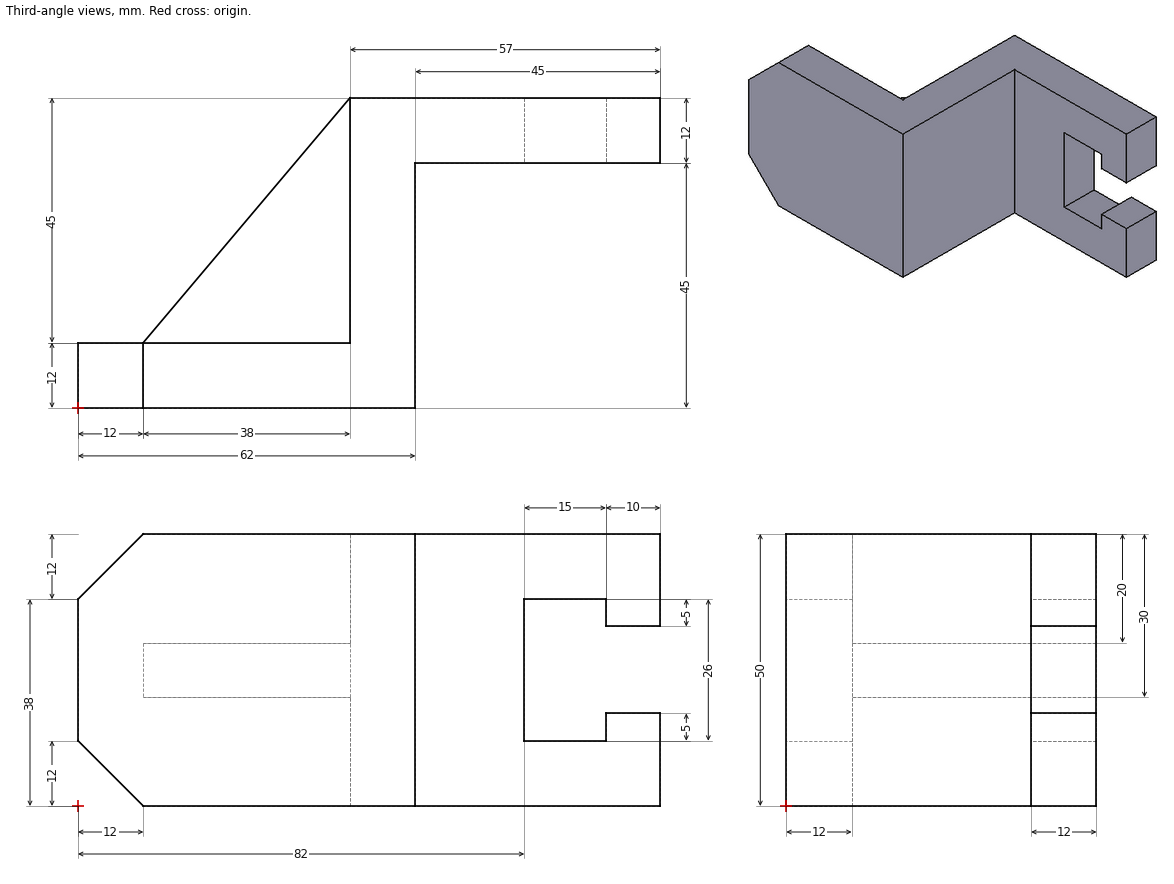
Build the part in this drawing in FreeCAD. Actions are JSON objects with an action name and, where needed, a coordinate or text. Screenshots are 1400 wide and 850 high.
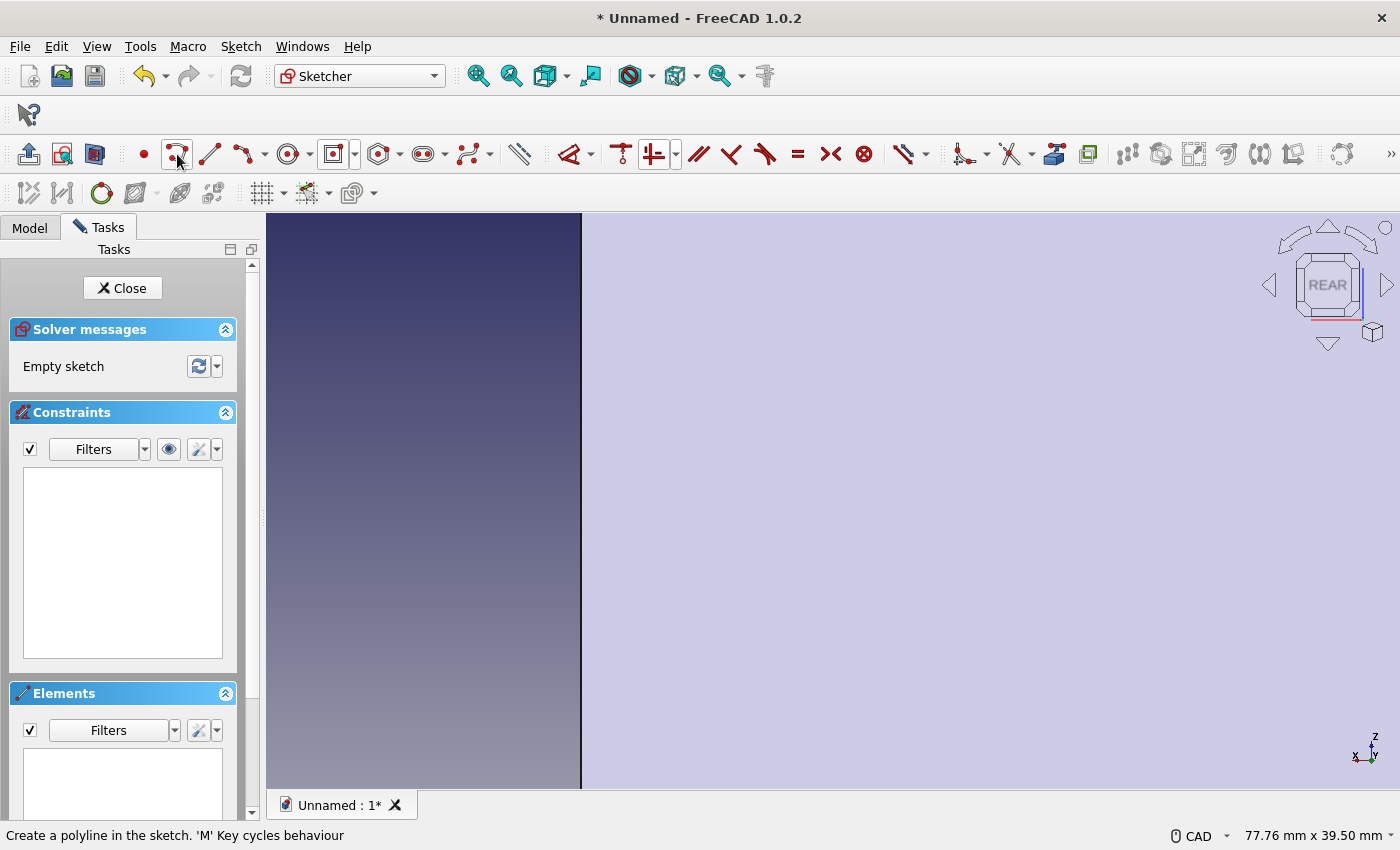
{"action": "left_click", "coordinate": [946, 689]}
{"action": "left_click", "coordinate": [946, 310]}
{"action": "left_click", "coordinate": [727, 310]}
{"action": "left_click", "coordinate": [727, 383]}
{"action": "left_click", "coordinate": [581, 383]}
{"action": "left_click", "coordinate": [581, 616]}
{"action": "left_click", "coordinate": [727, 616]}
{"action": "left_click", "coordinate": [727, 689]}
{"action": "left_click", "coordinate": [946, 690]}
{"action": "key", "text": "Escape"}
{"action": "key", "text": "Escape"}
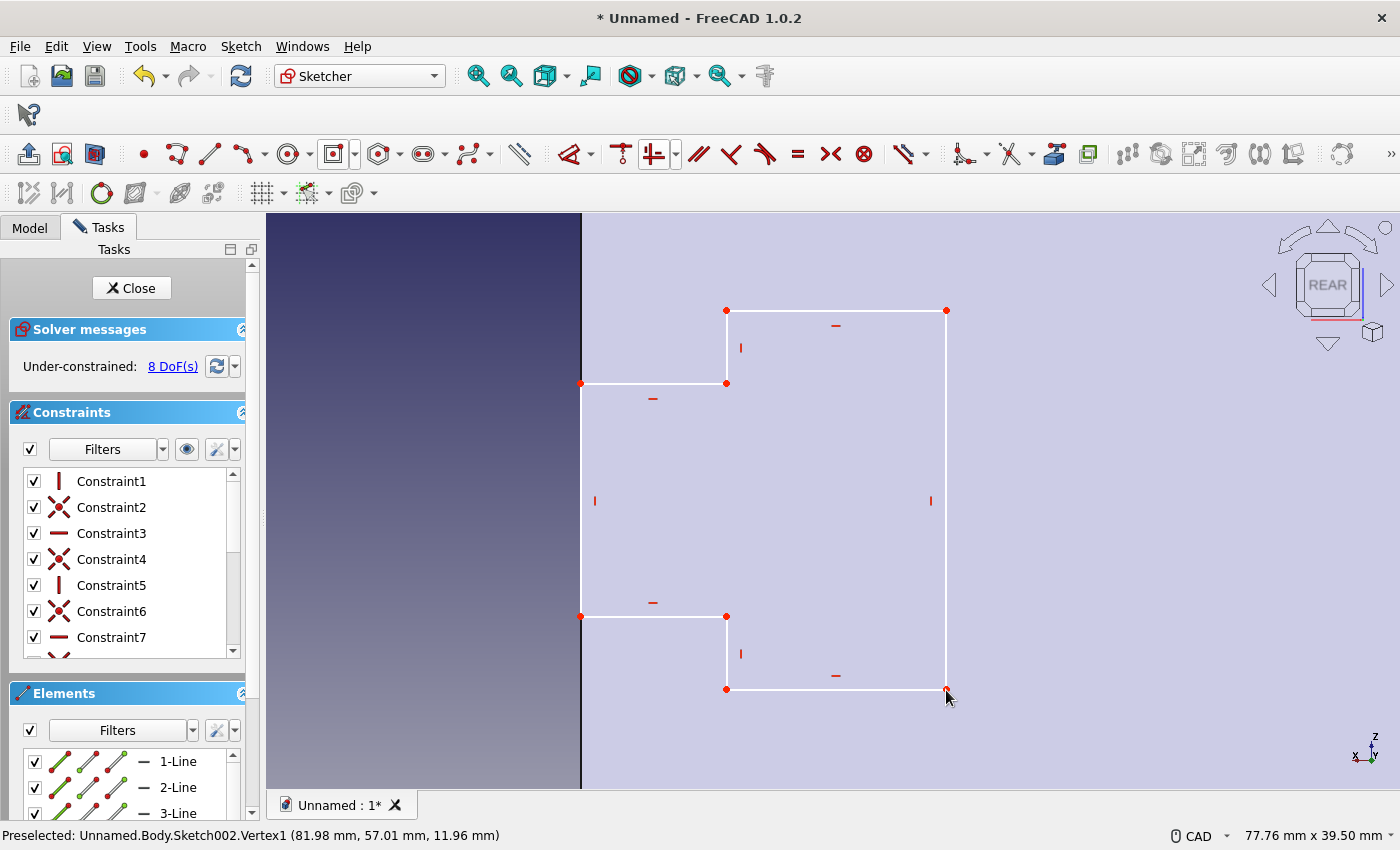
{"action": "left_click", "coordinate": [568, 154]}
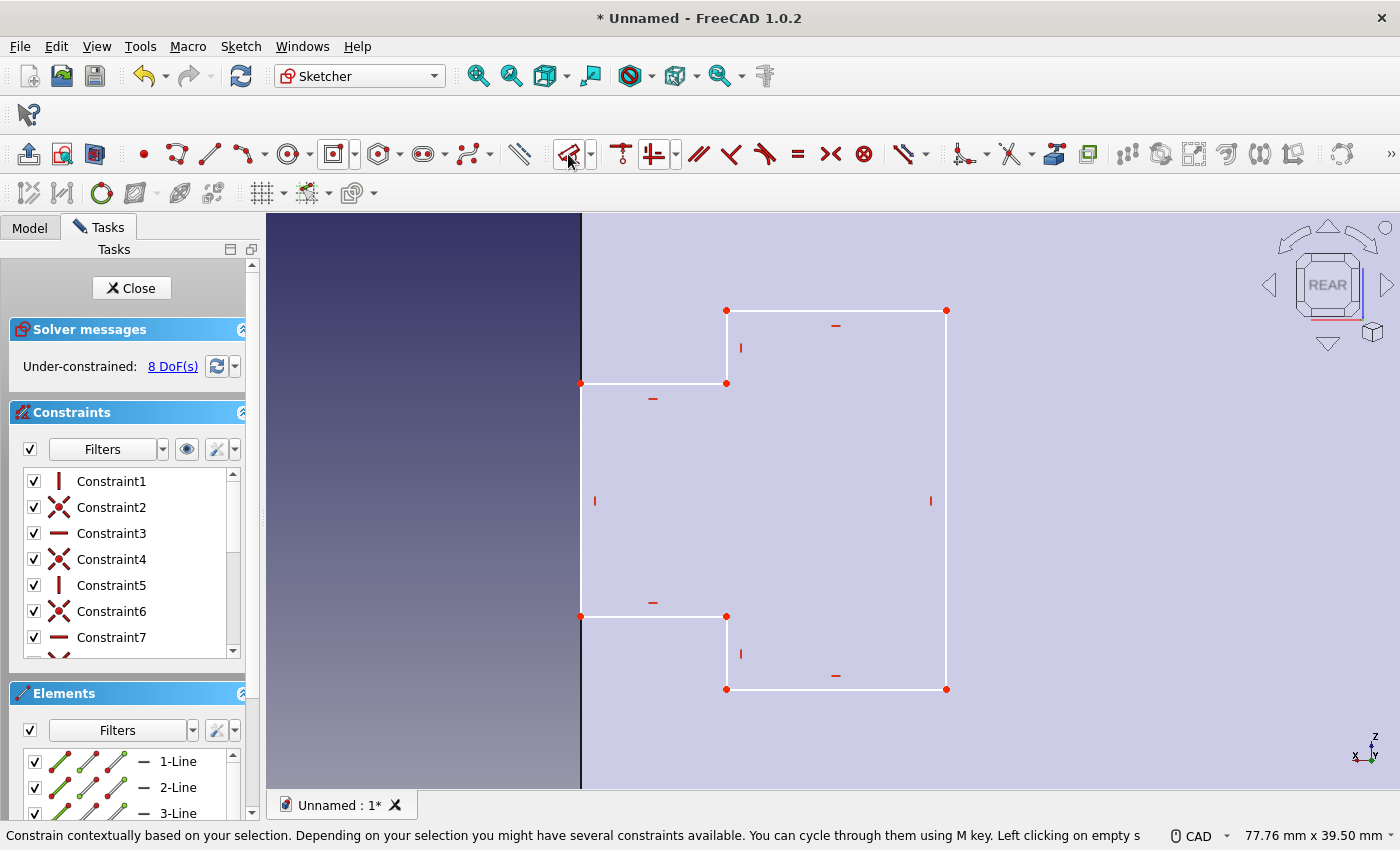
{"action": "left_click", "coordinate": [727, 333]}
{"action": "left_click", "coordinate": [693, 347]}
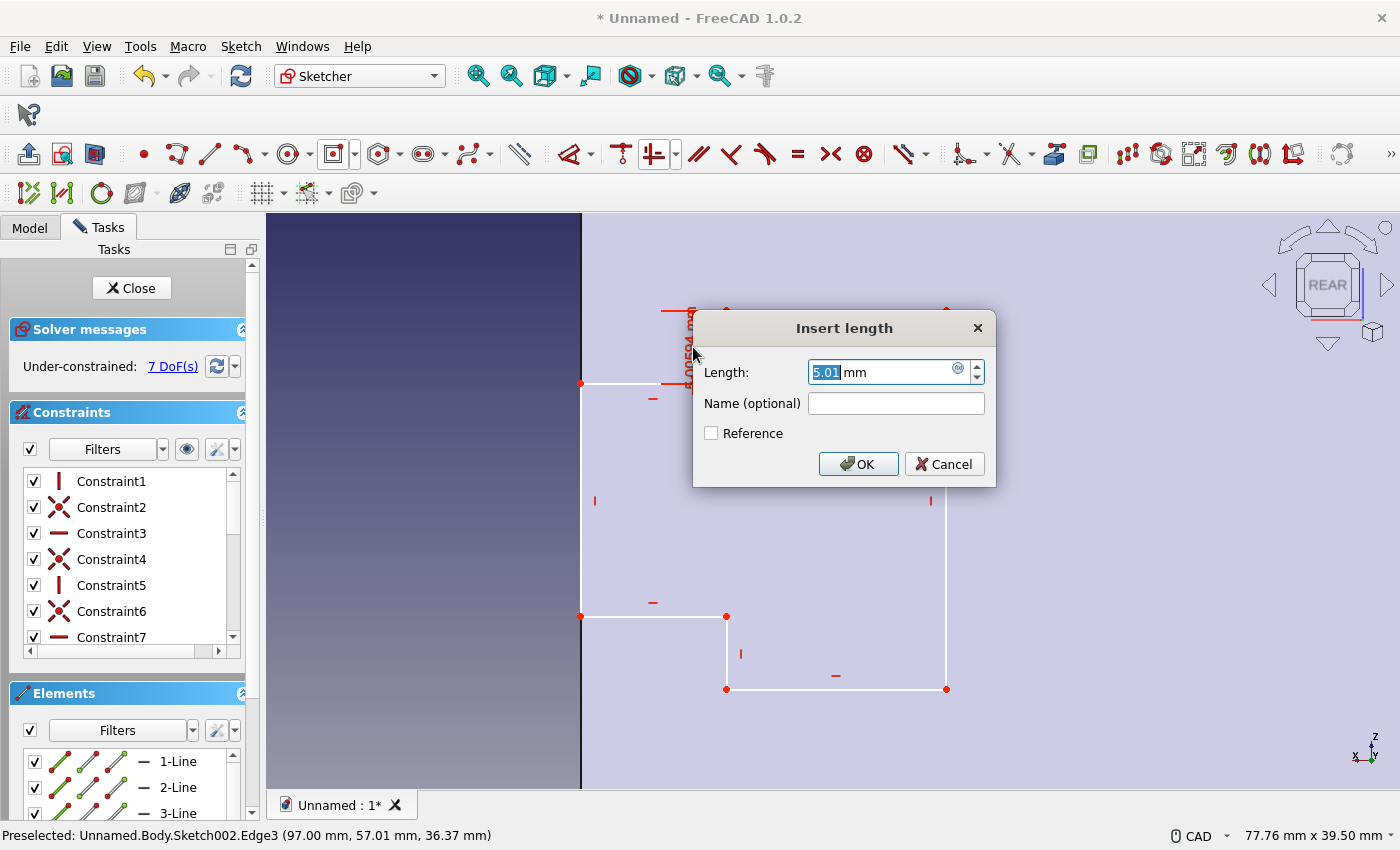
{"action": "type", "text": "5"}
{"action": "key", "text": "Return"}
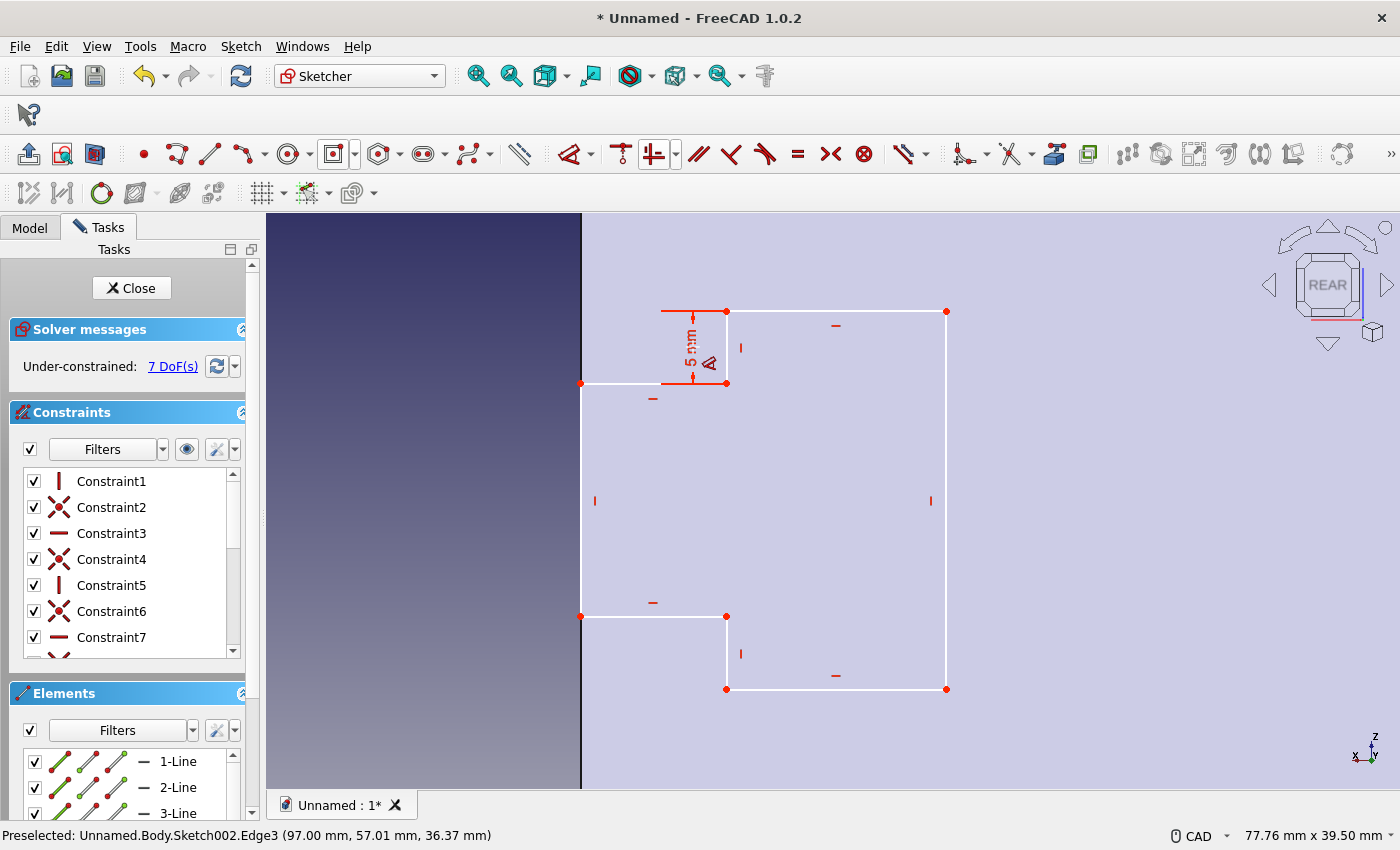
{"action": "left_click", "coordinate": [727, 639]}
{"action": "left_click", "coordinate": [693, 653]}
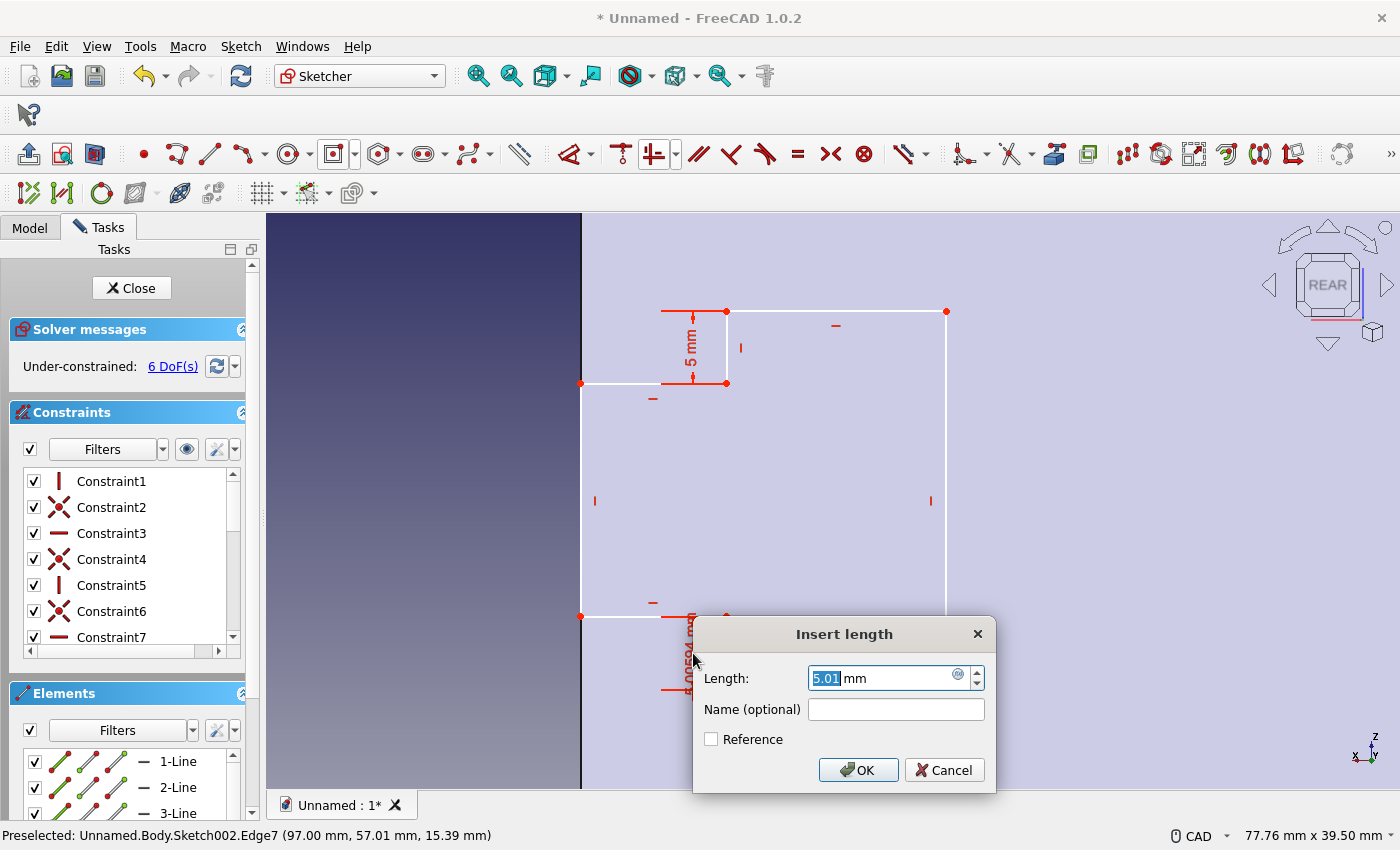
{"action": "type", "text": "5"}
{"action": "key", "text": "Return"}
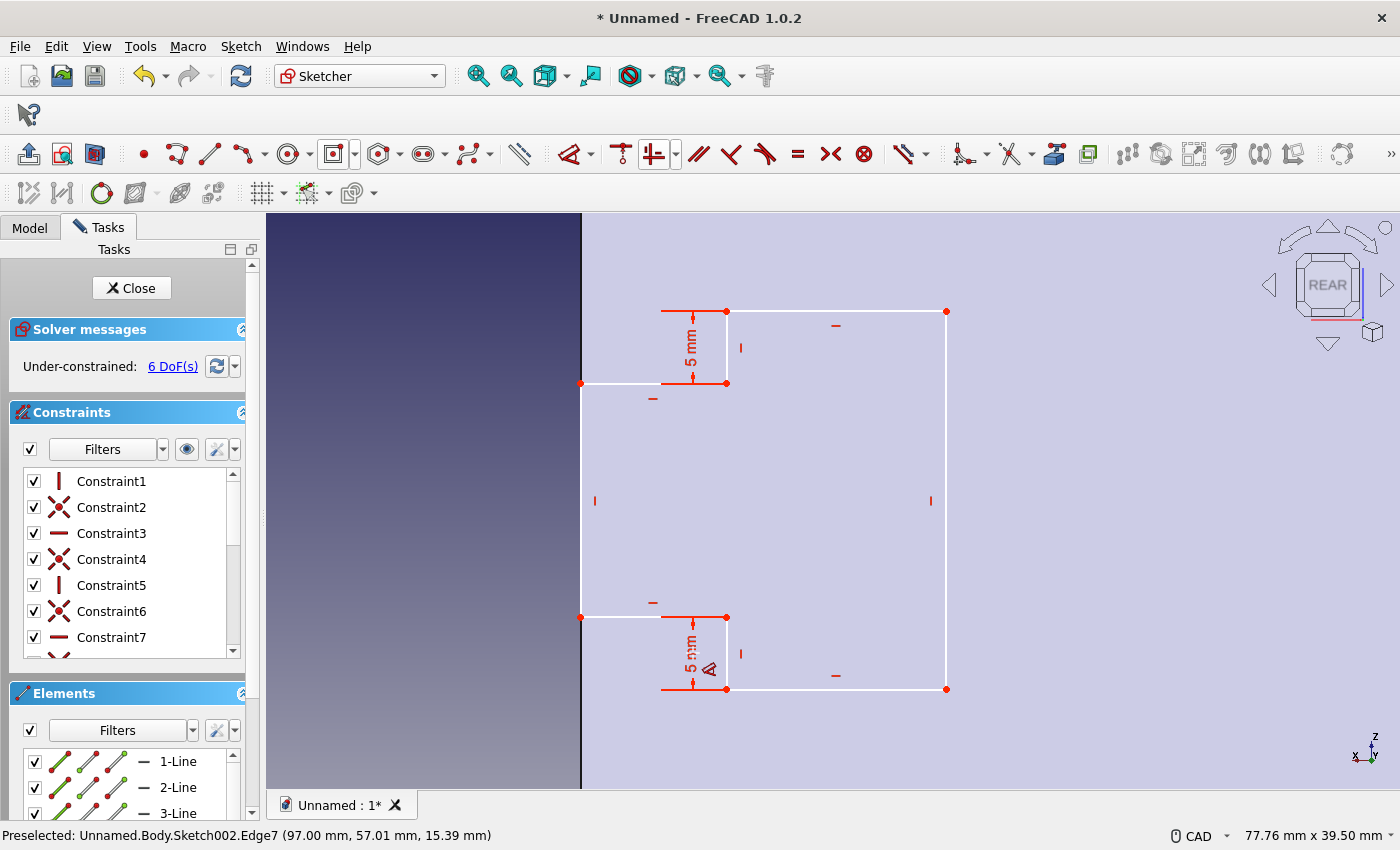
{"action": "left_click", "coordinate": [946, 576]}
{"action": "left_click", "coordinate": [980, 501]}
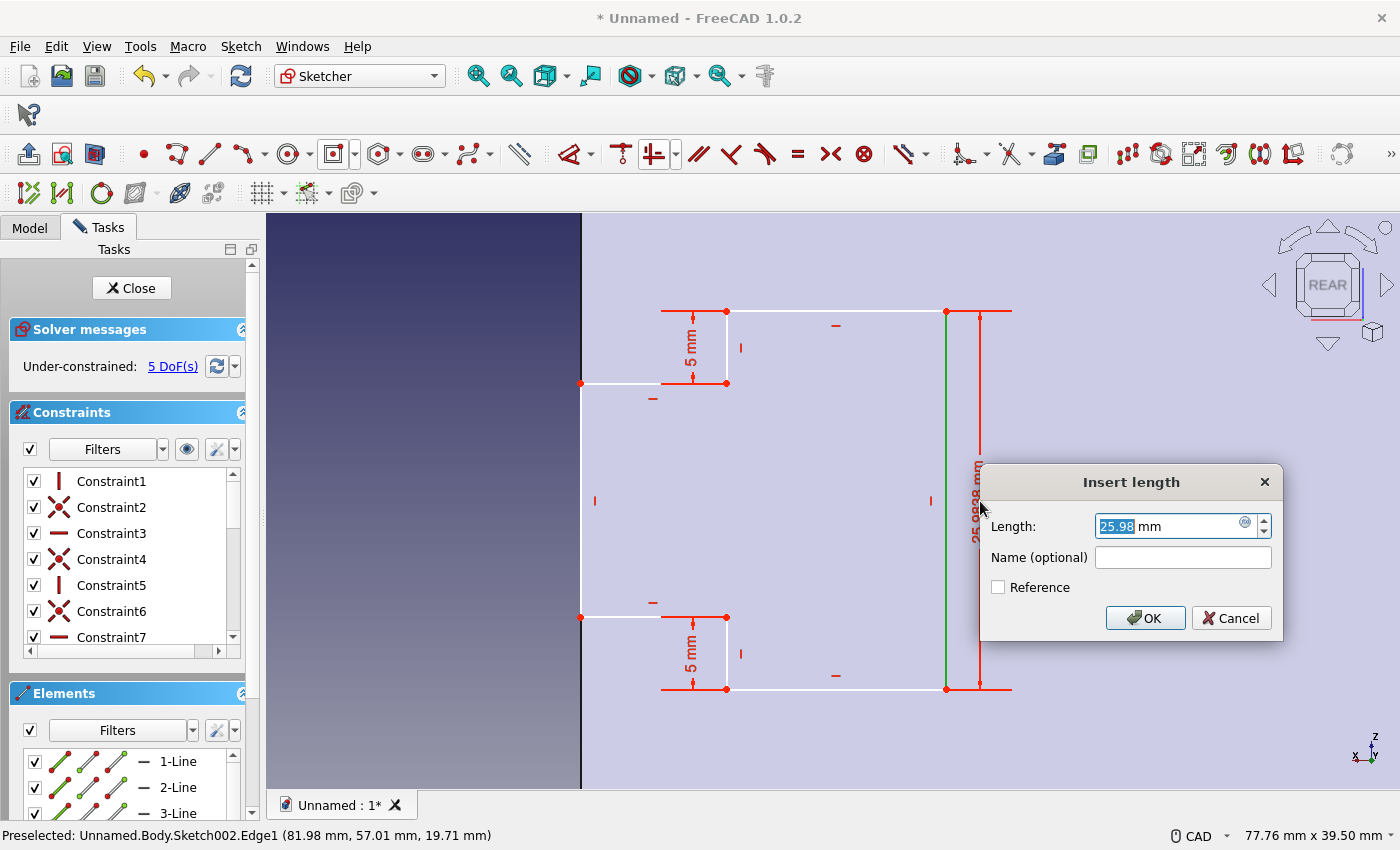
{"action": "type", "text": "26"}
{"action": "key", "text": "Return"}